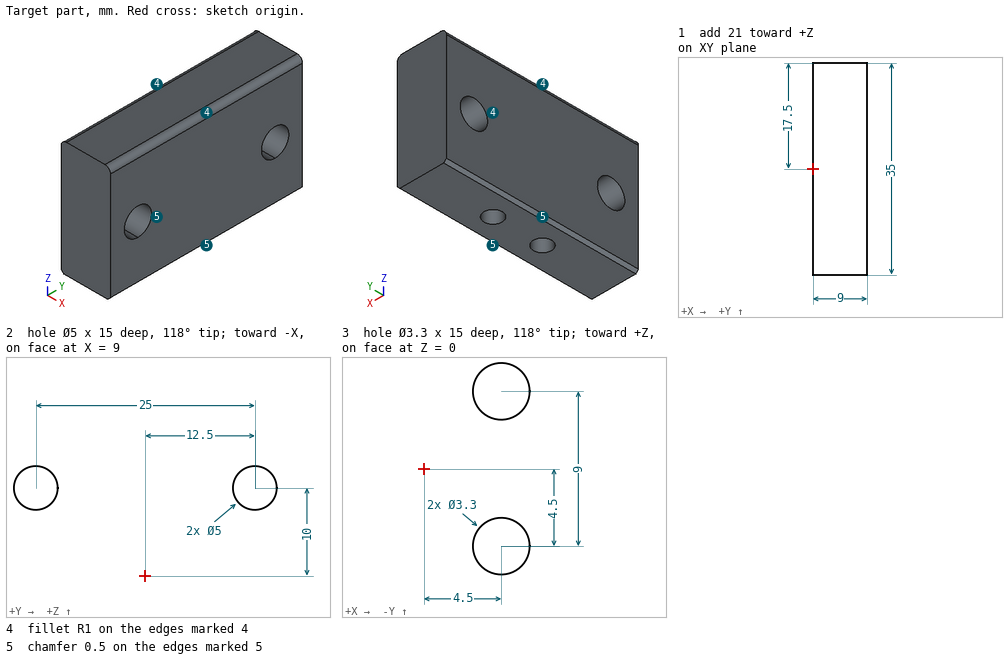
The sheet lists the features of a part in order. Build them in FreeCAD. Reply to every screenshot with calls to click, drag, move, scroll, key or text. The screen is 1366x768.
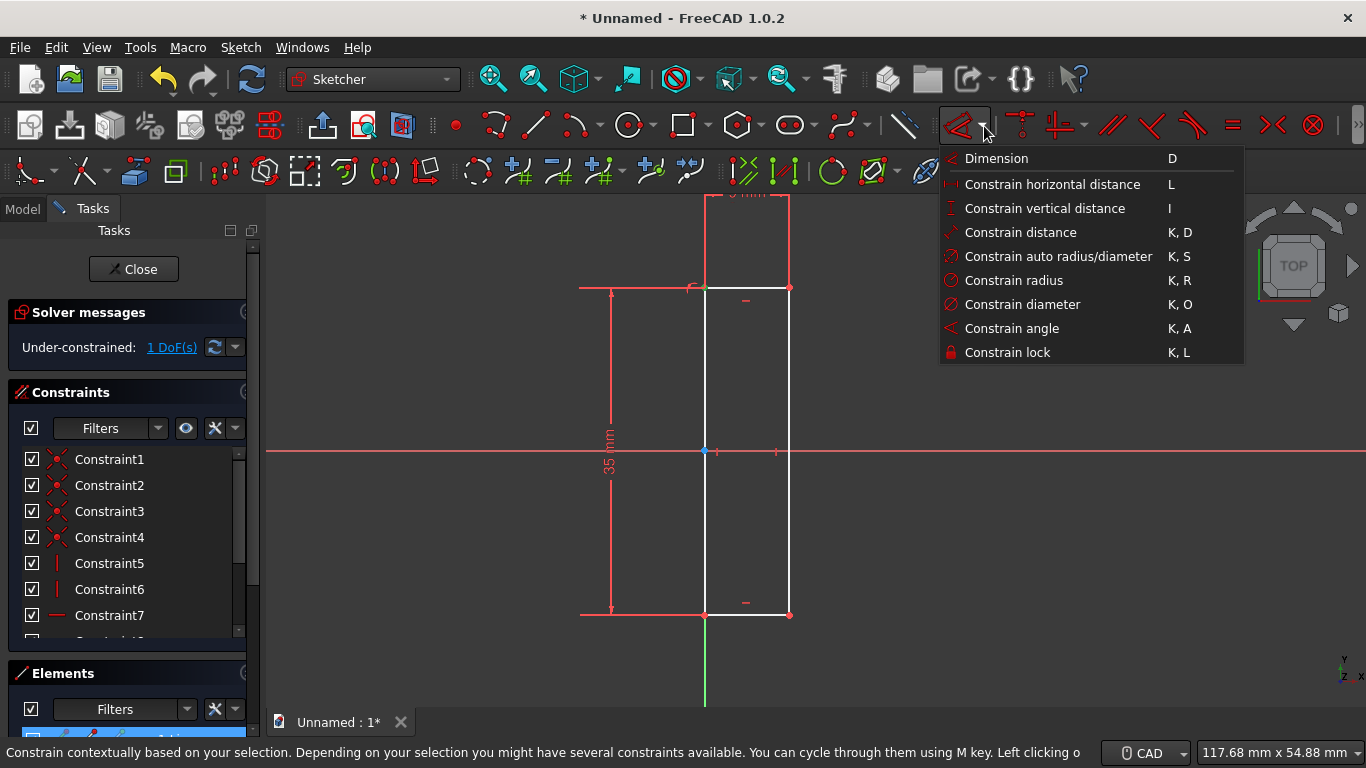
click(1092, 208)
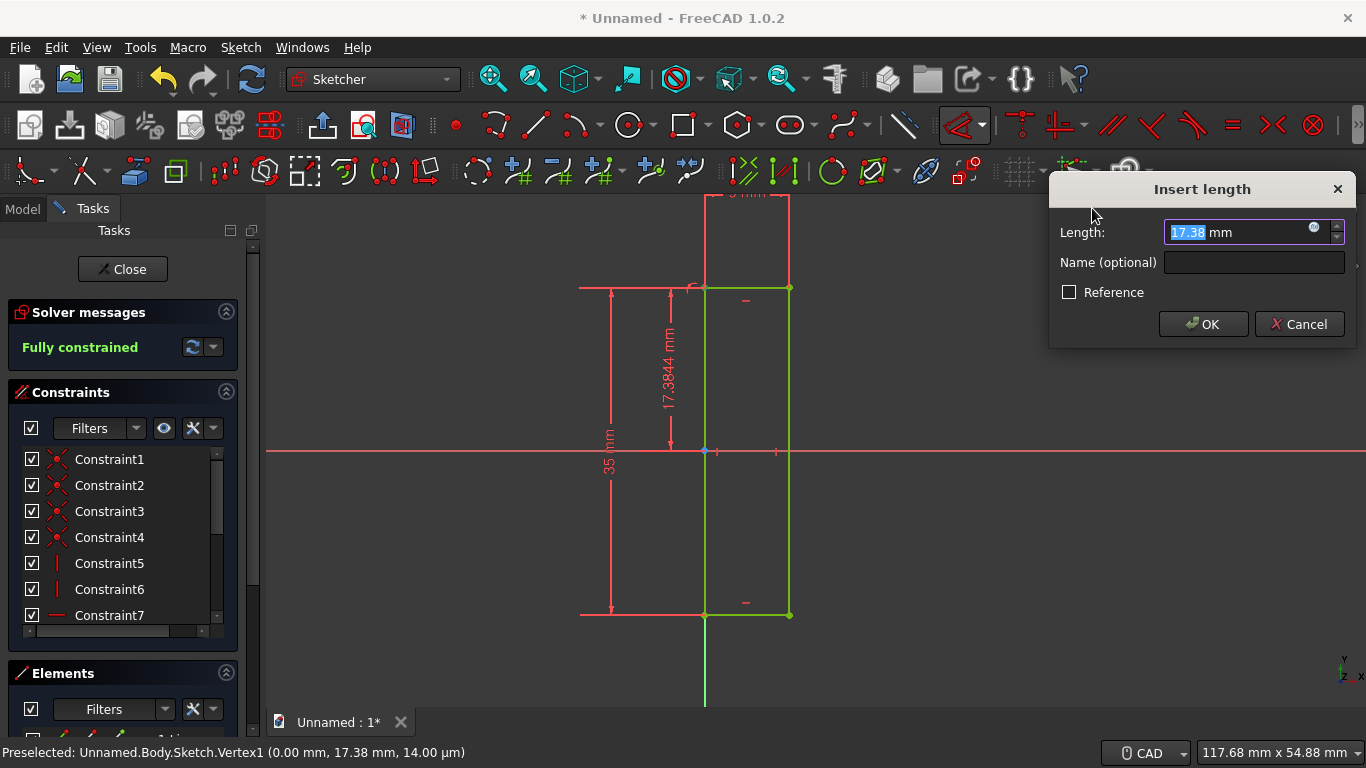
text(17.5)
key(Return)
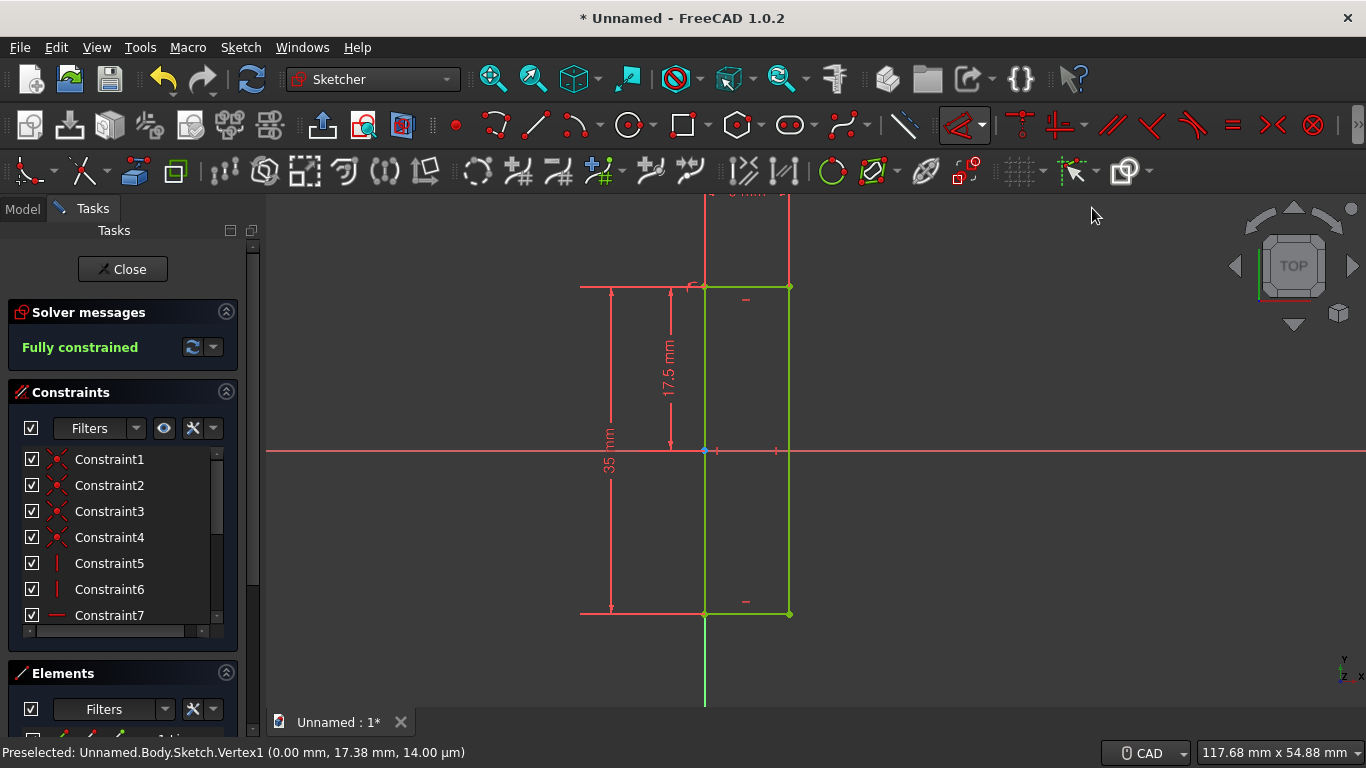
click(123, 269)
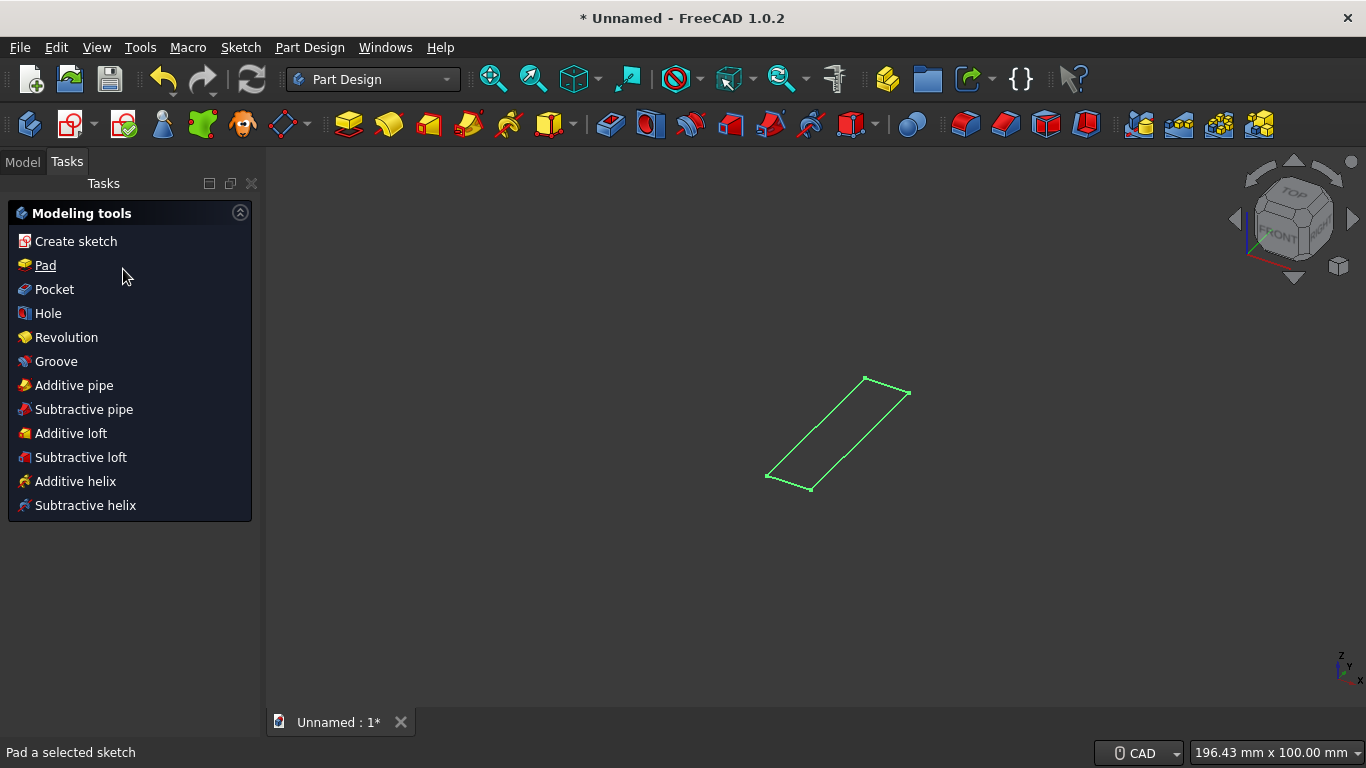
click(350, 124)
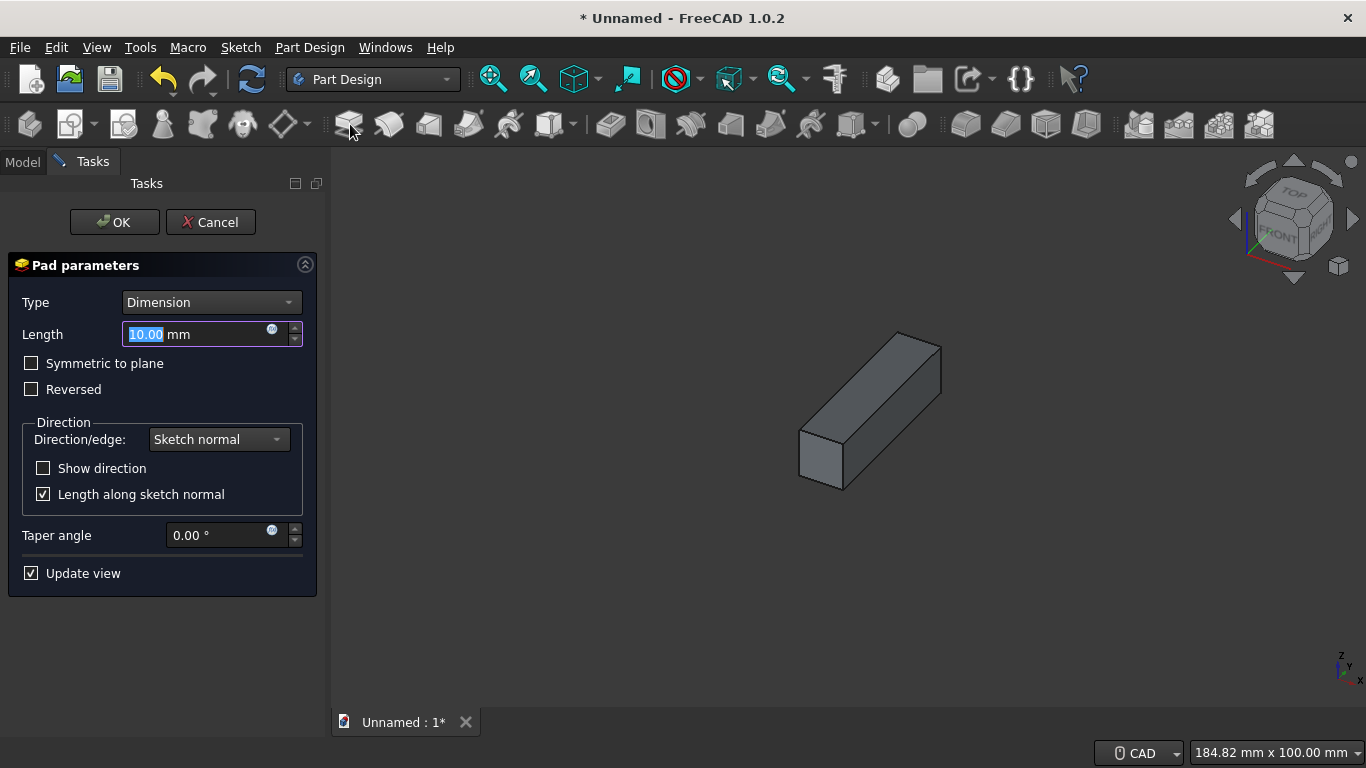
text(21)
key(Tab)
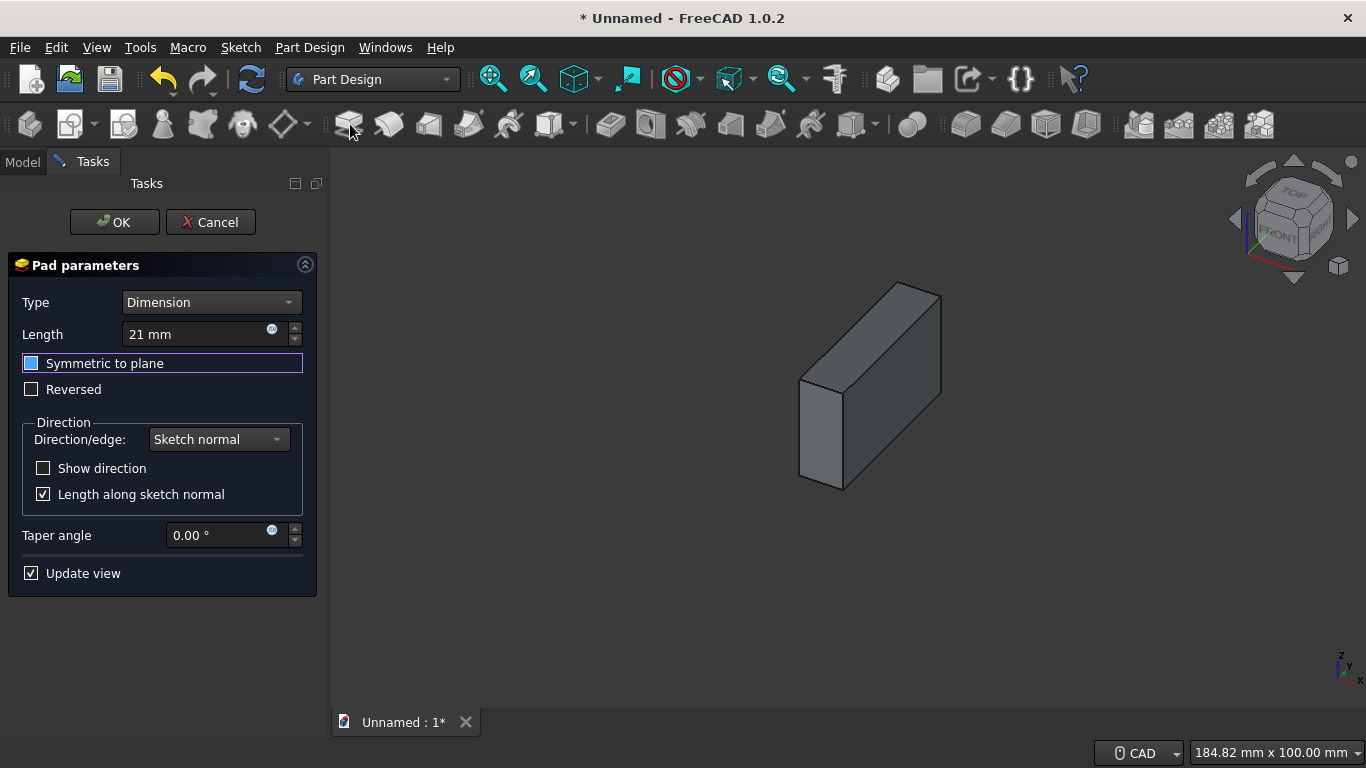
click(115, 222)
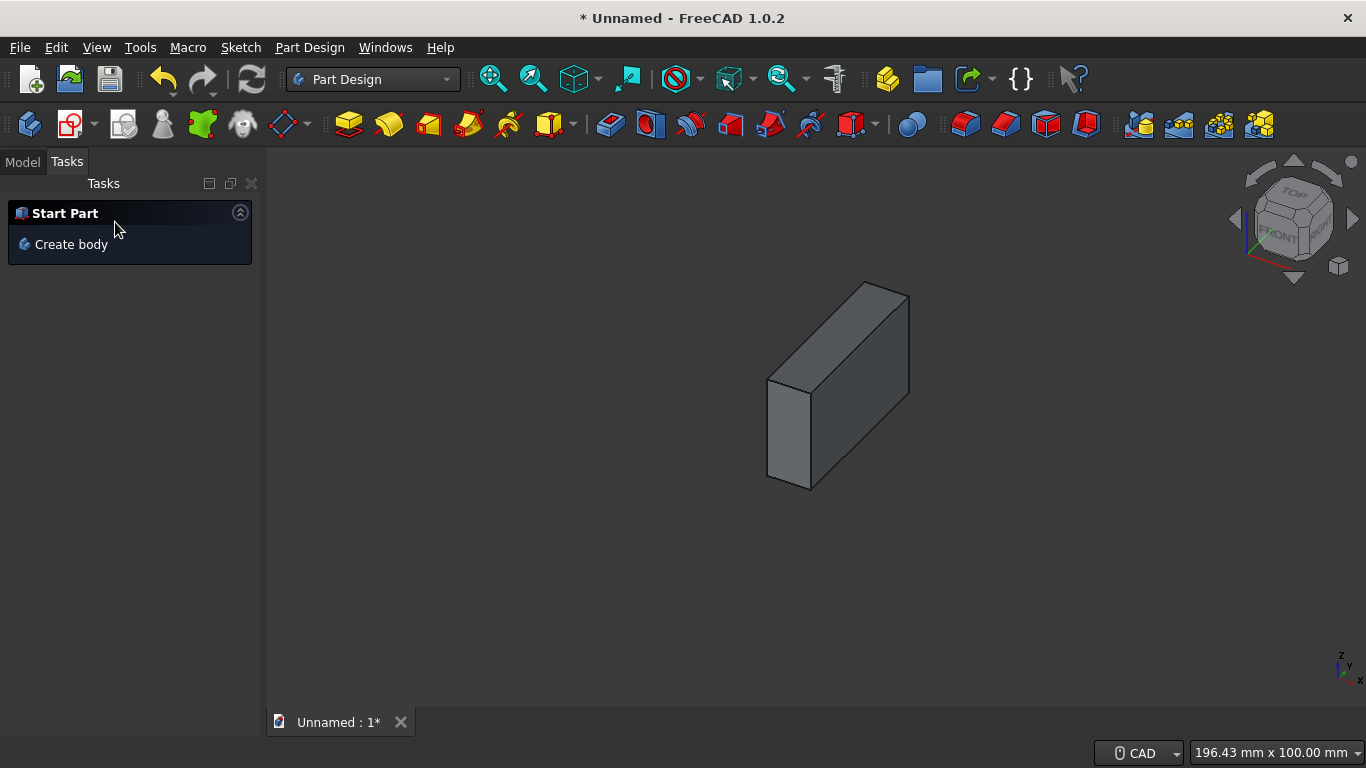
key(v)
key(f)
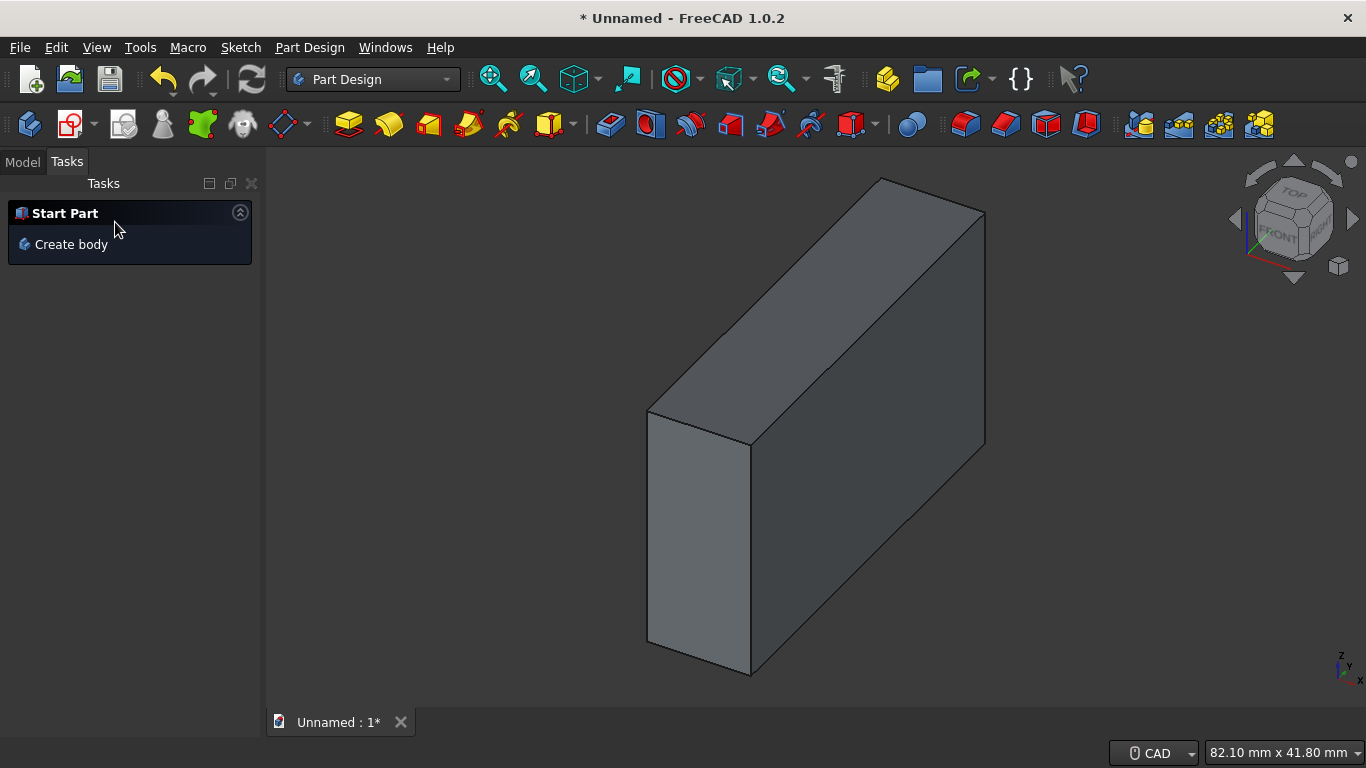
click(902, 410)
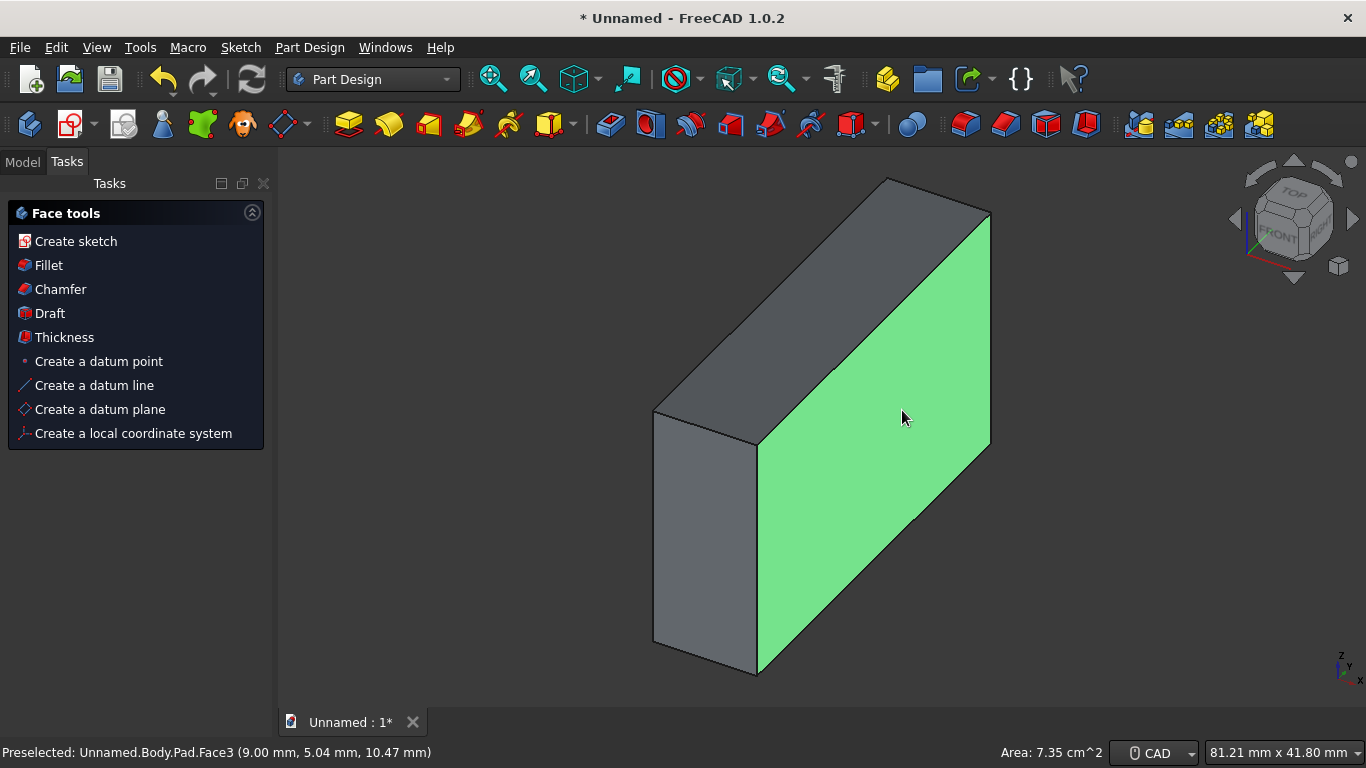
click(70, 124)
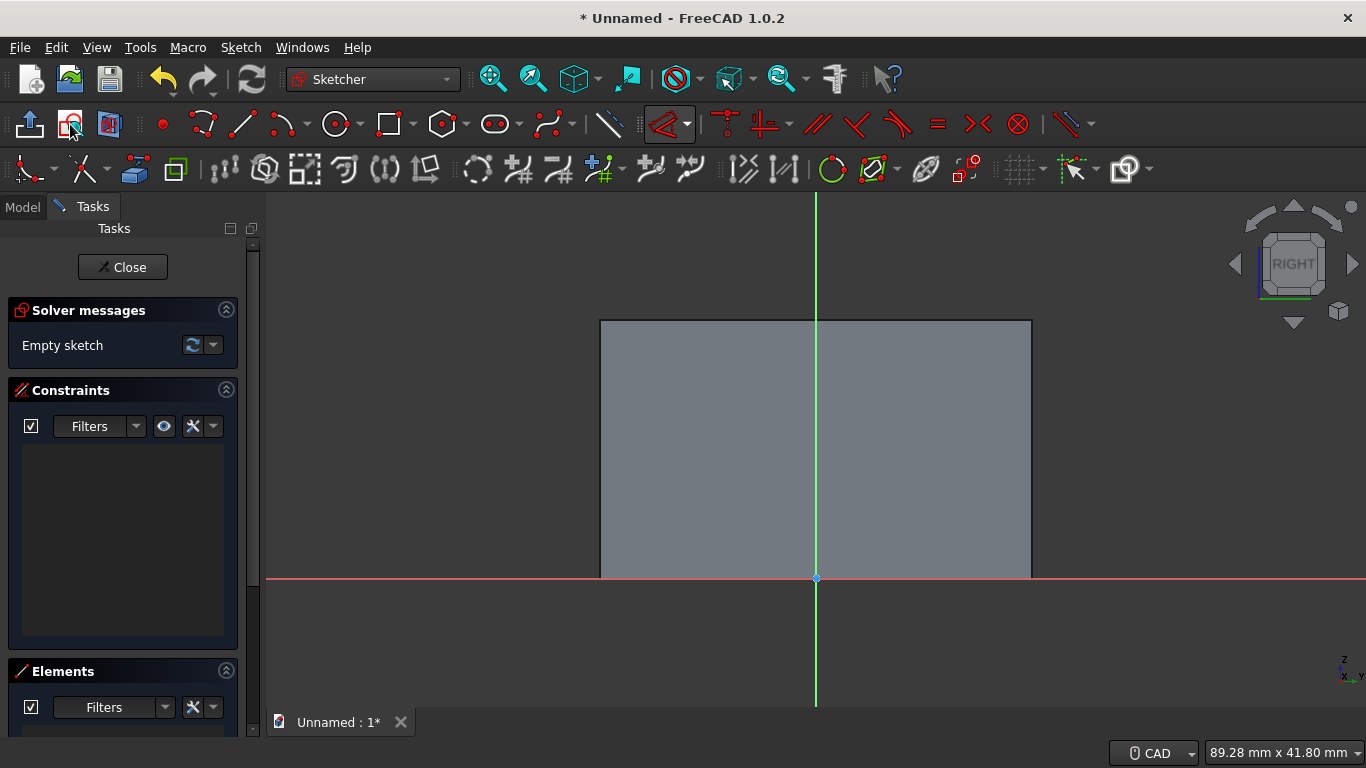
scroll(899, 566, up, 3)